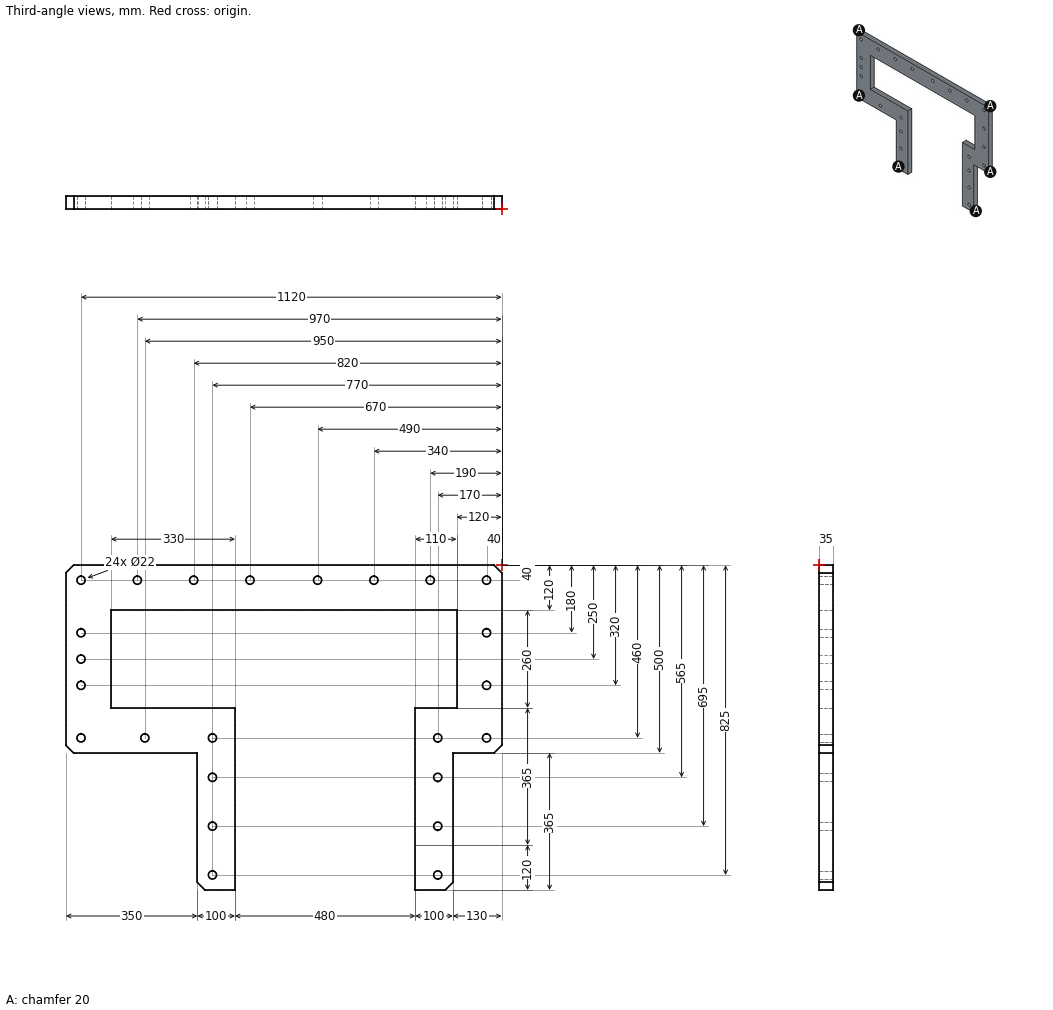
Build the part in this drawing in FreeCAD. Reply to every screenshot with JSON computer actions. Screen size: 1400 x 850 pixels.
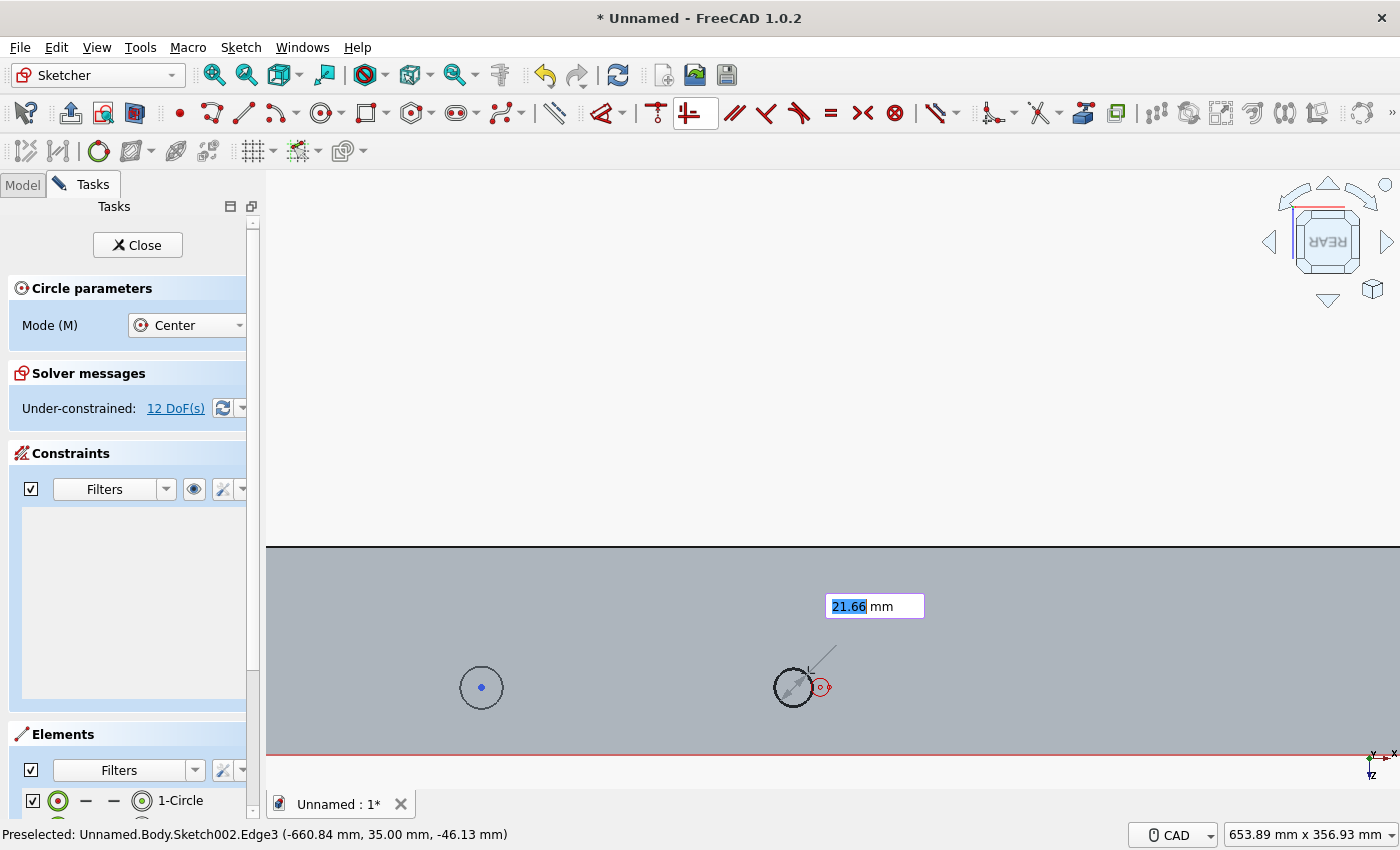
{"action": "left_click", "coordinate": [808, 672]}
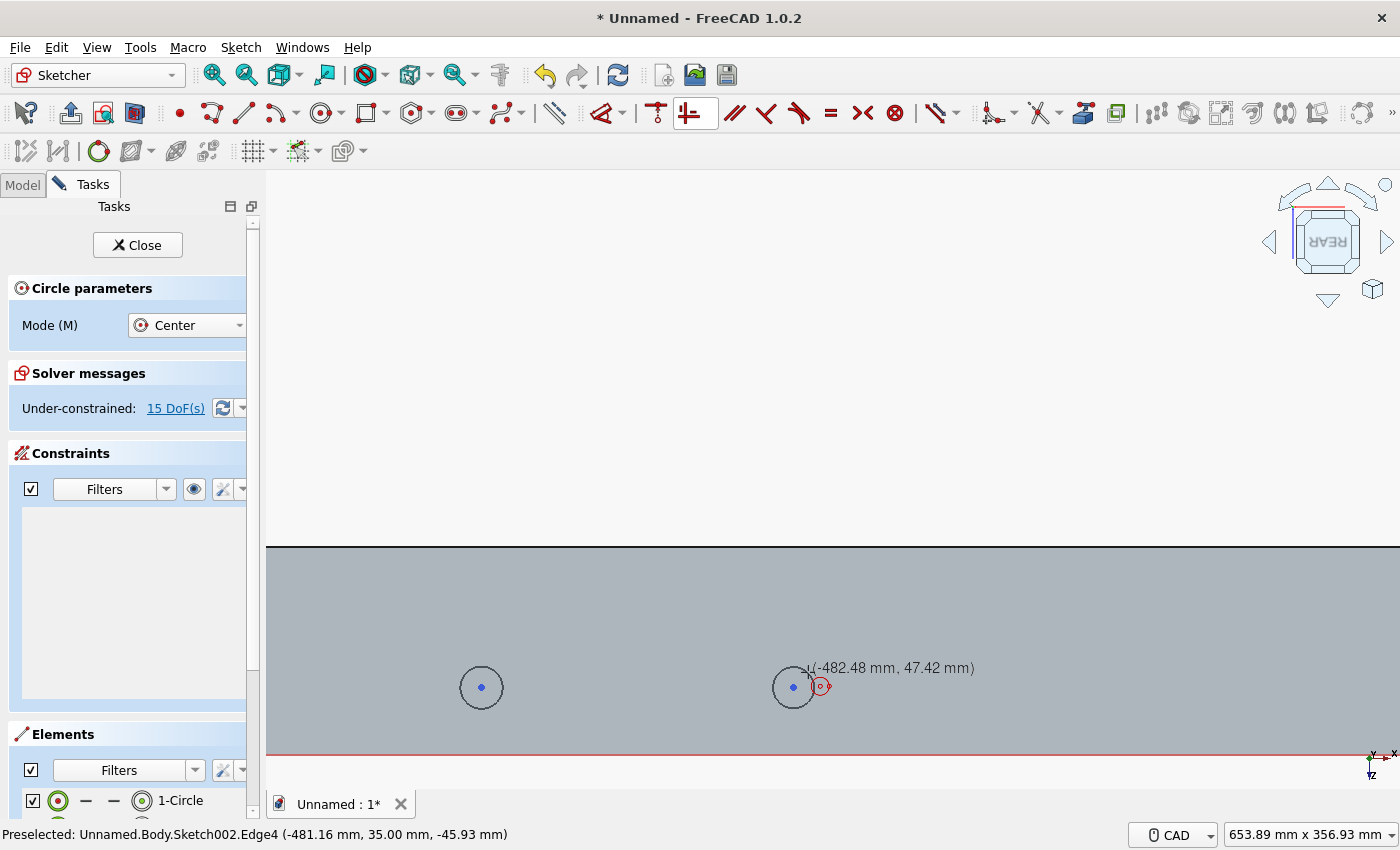
{"action": "scroll", "coordinate": [808, 673], "scroll_direction": "down", "scroll_amount": 6}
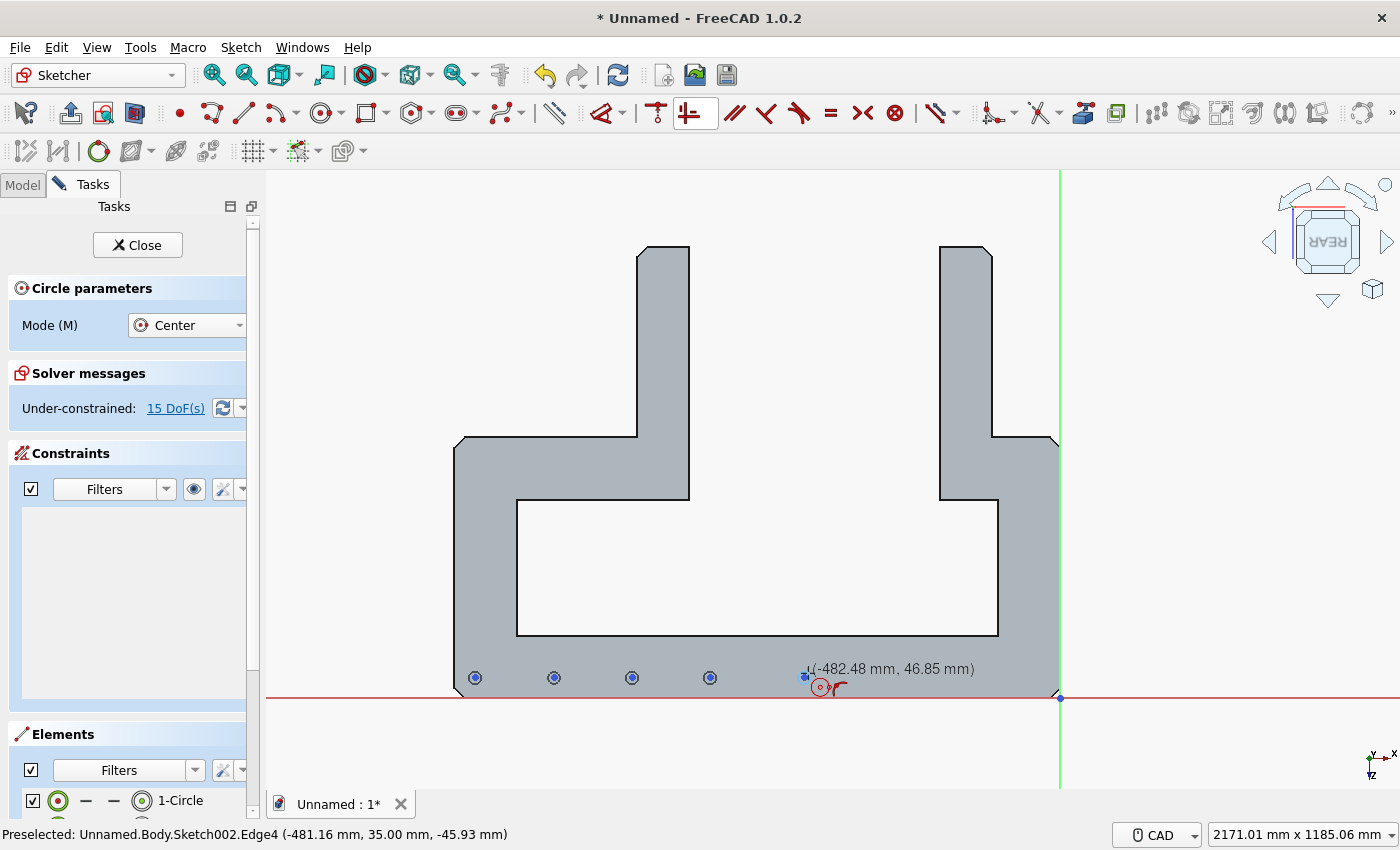
{"action": "left_click", "coordinate": [883, 677]}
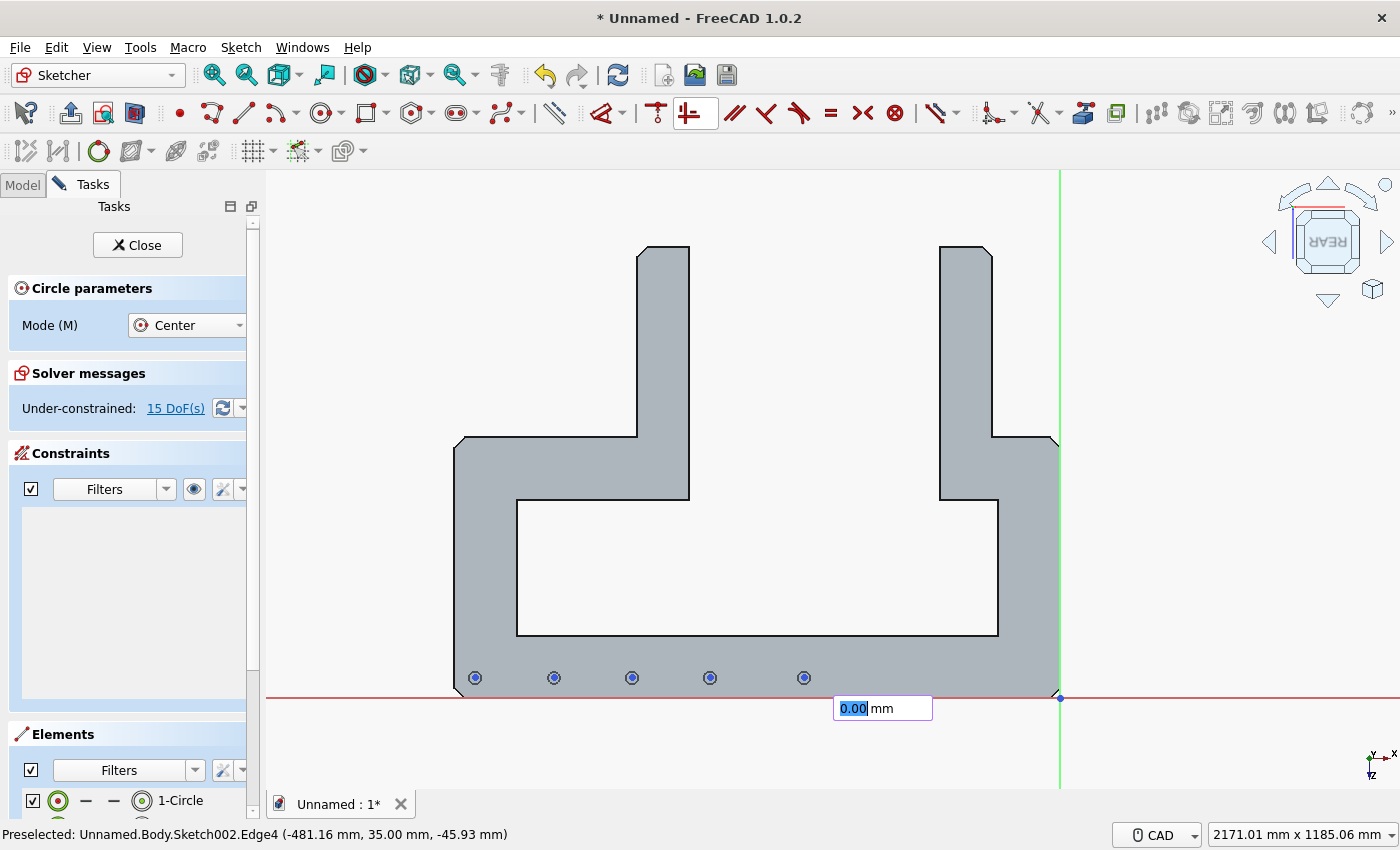
{"action": "scroll", "coordinate": [887, 673], "scroll_direction": "up", "scroll_amount": 6}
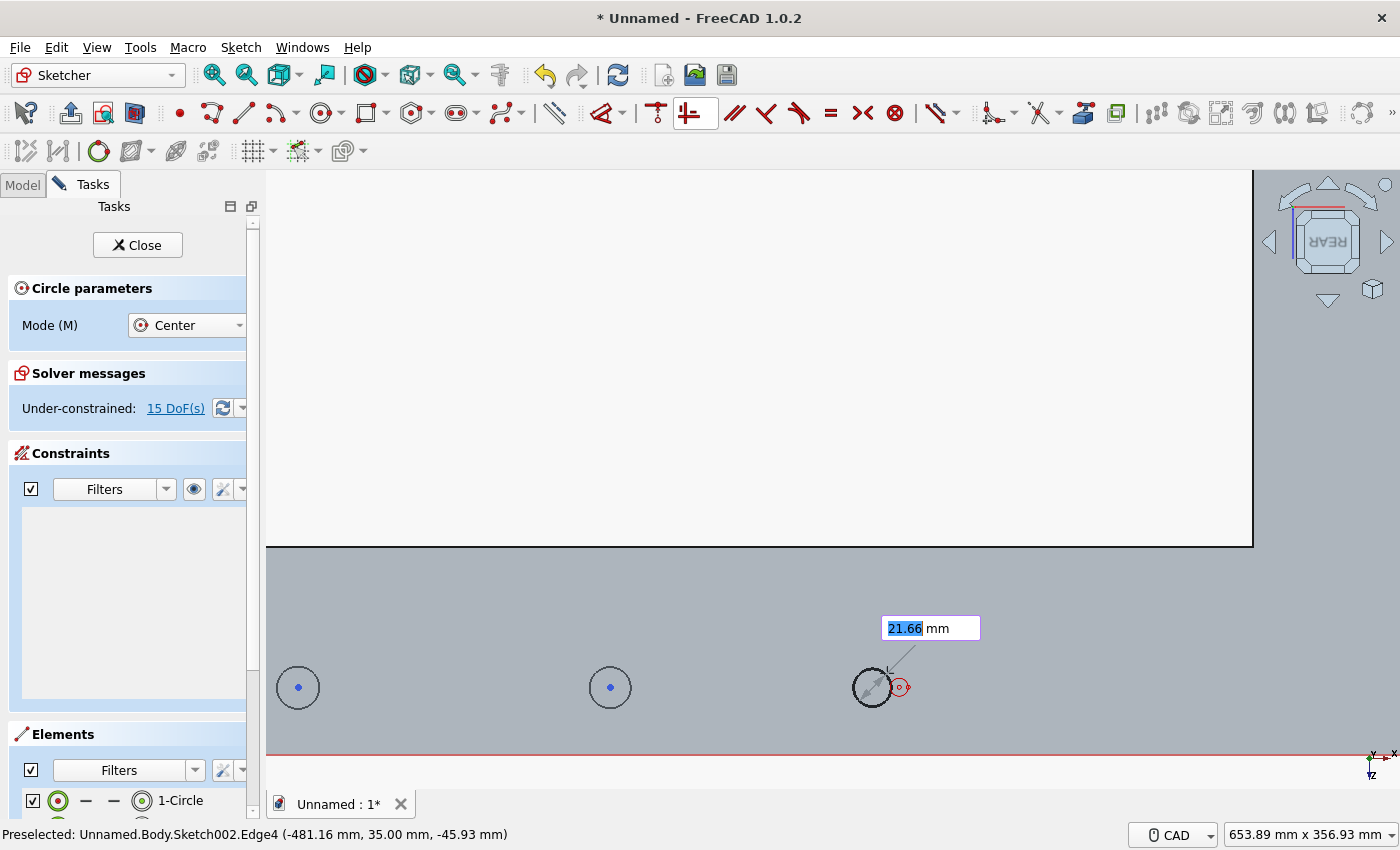
{"action": "left_click", "coordinate": [885, 672]}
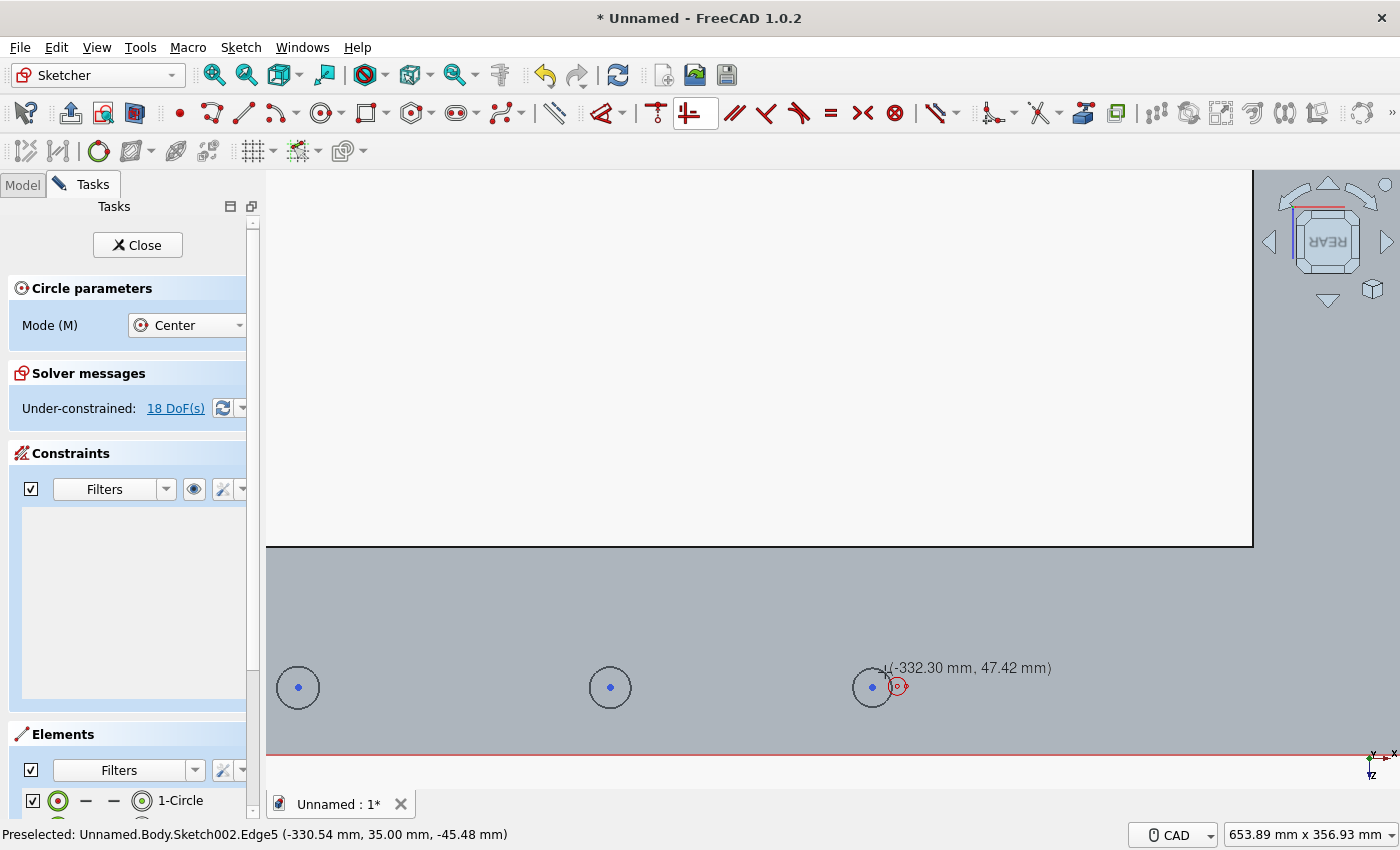
{"action": "scroll", "coordinate": [887, 673], "scroll_direction": "down", "scroll_amount": 6}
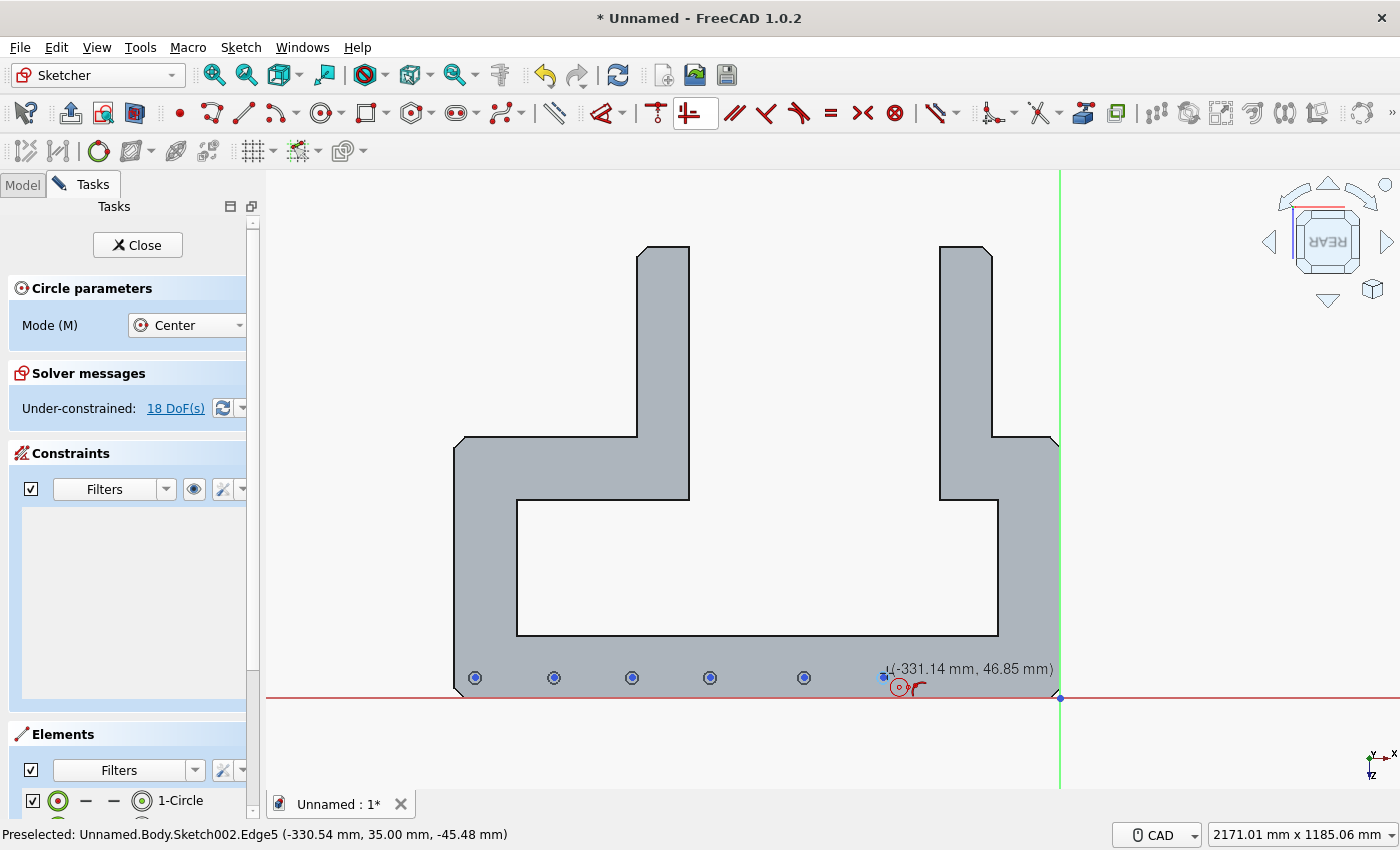
{"action": "left_click", "coordinate": [961, 677]}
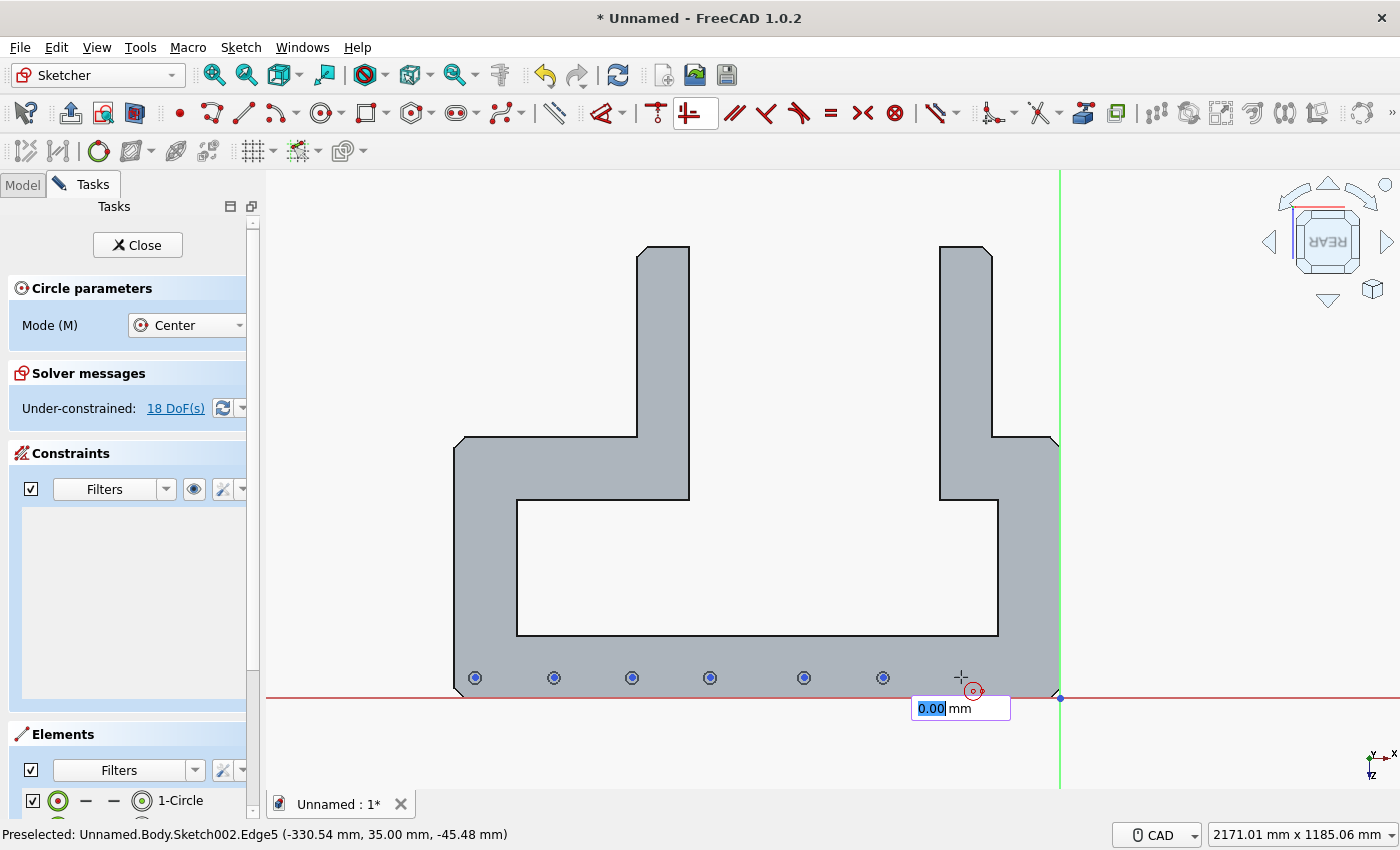
{"action": "scroll", "coordinate": [965, 673], "scroll_direction": "up", "scroll_amount": 6}